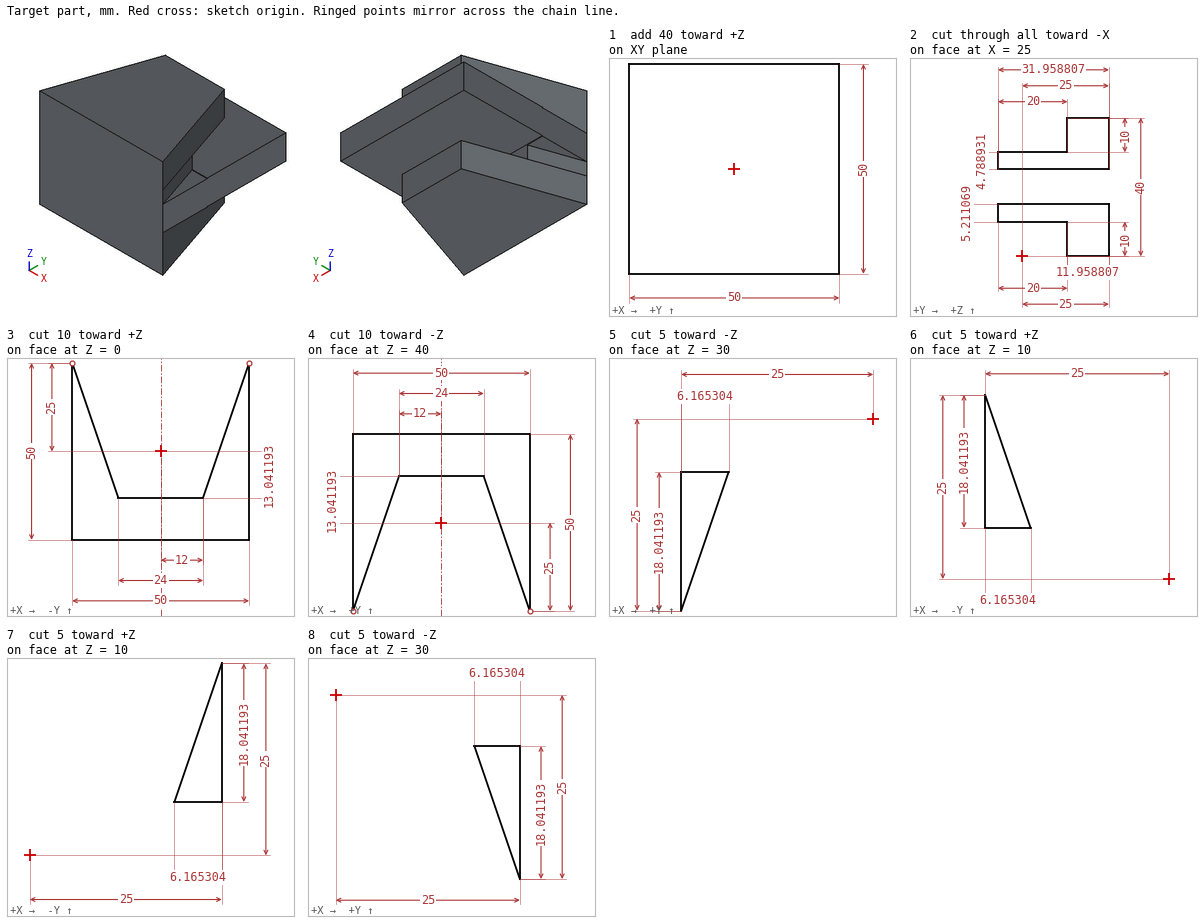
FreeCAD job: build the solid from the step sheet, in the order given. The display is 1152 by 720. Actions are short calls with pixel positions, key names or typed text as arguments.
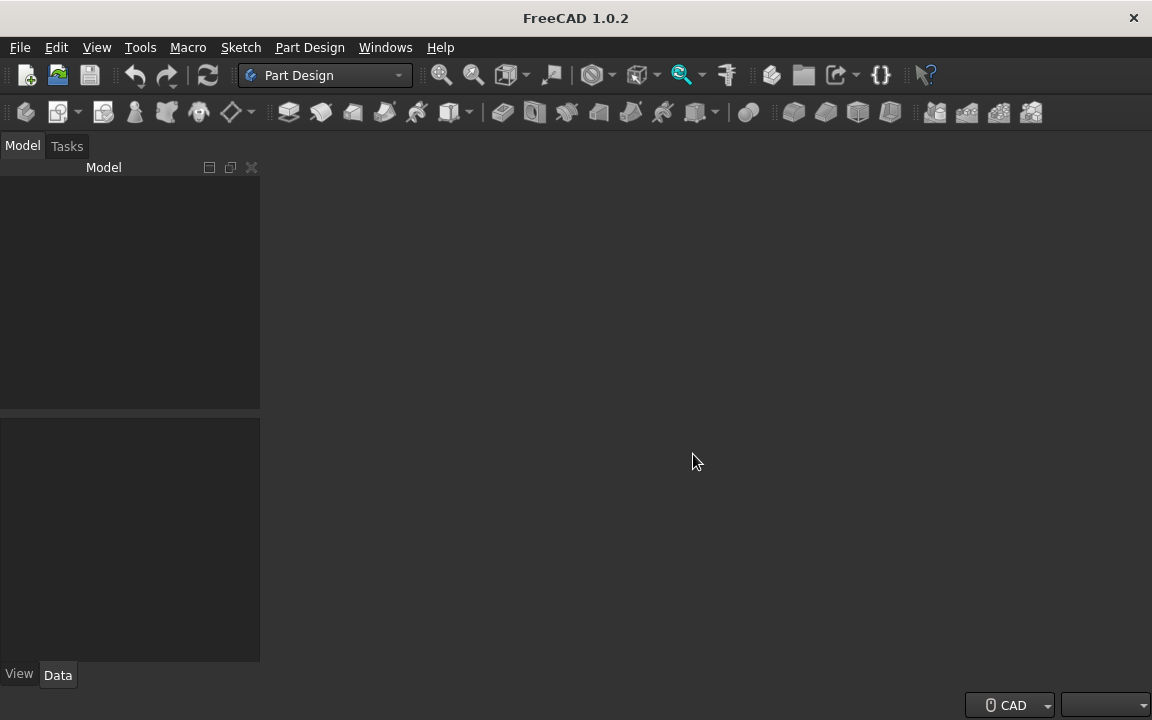
key(ctrl+n)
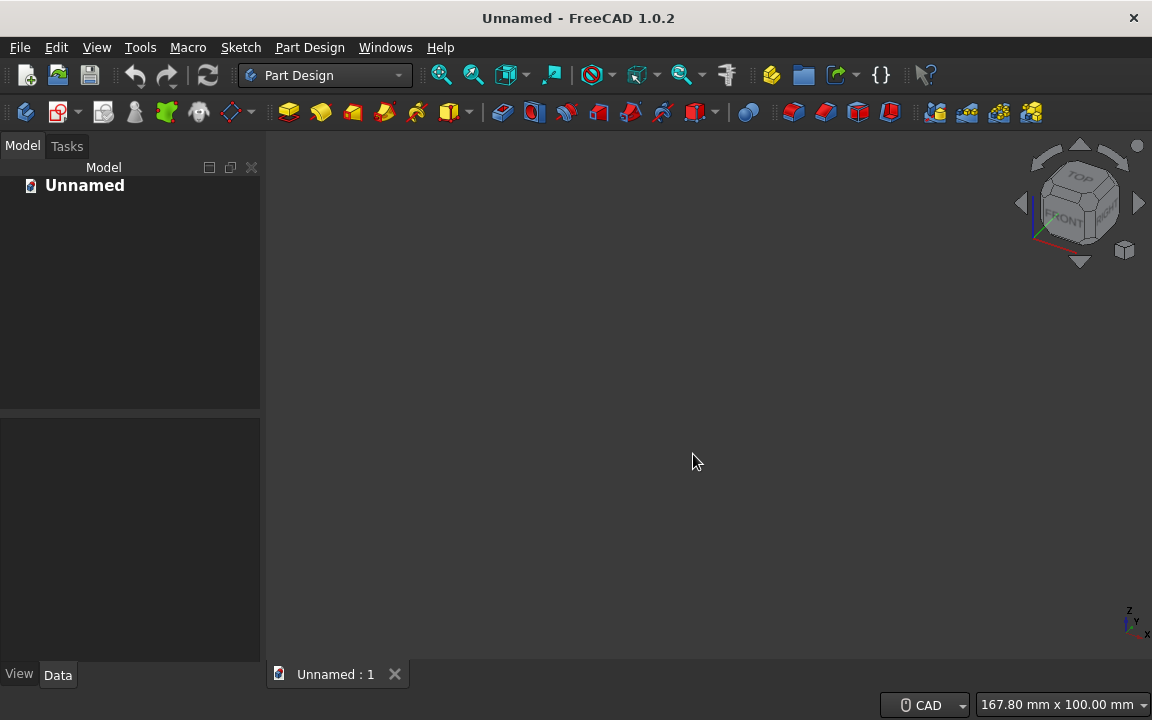
click(58, 112)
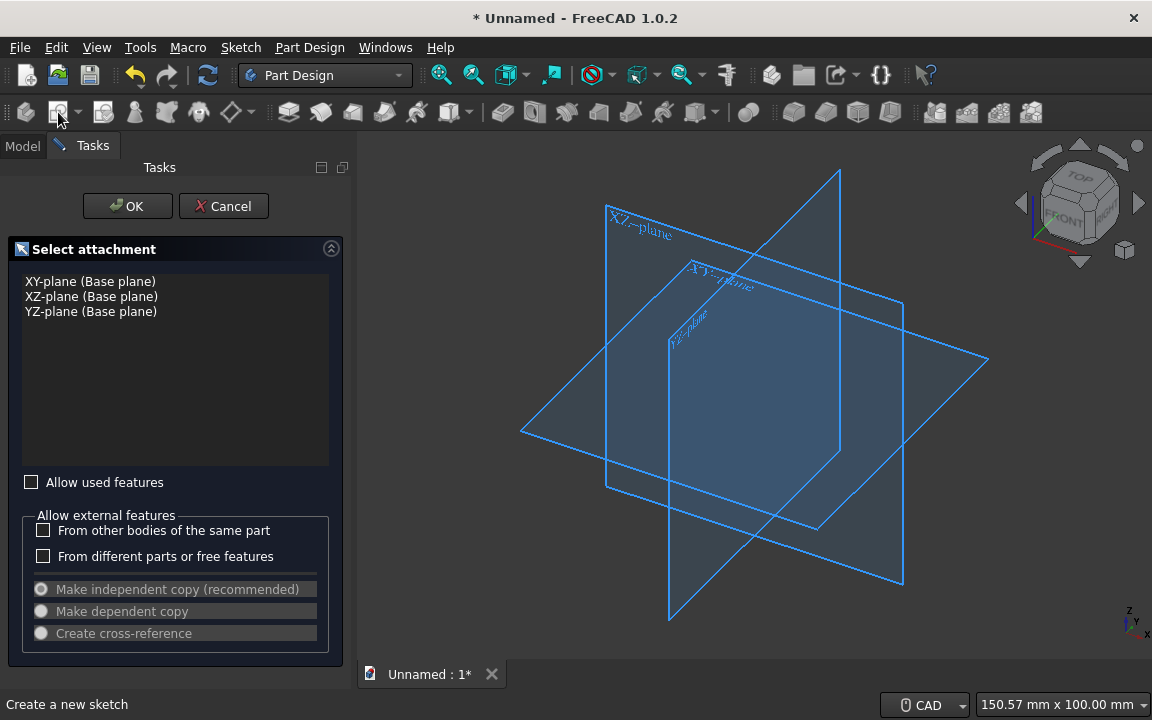
click(82, 282)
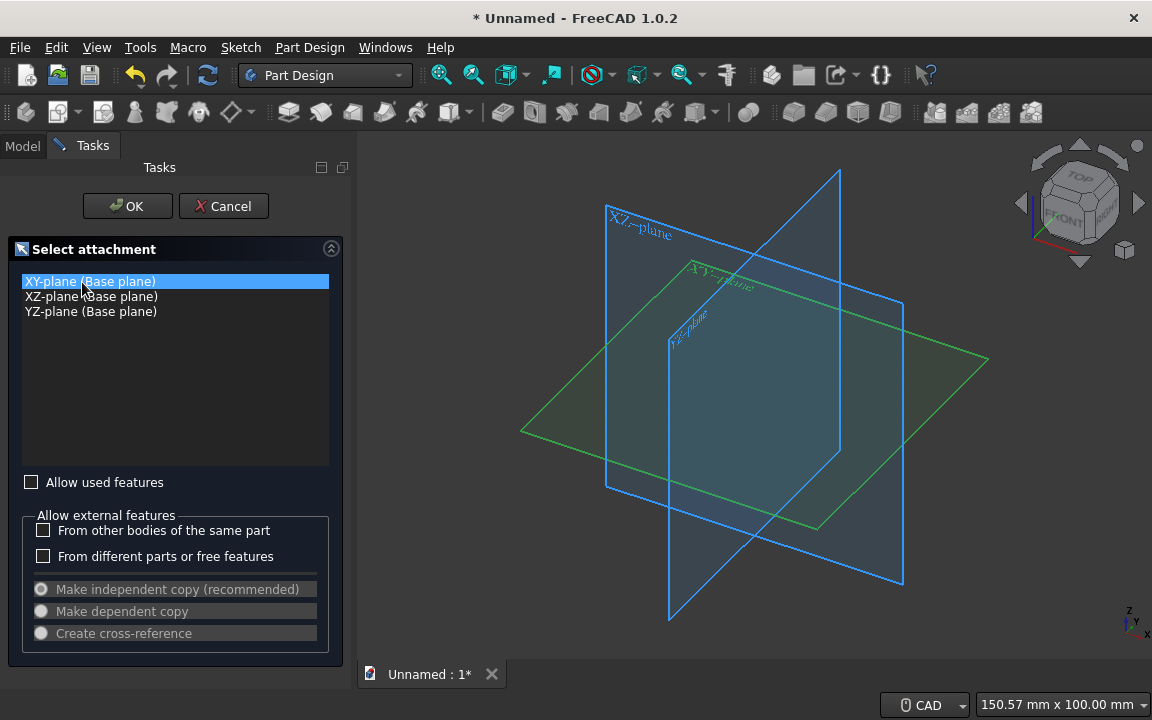
click(128, 206)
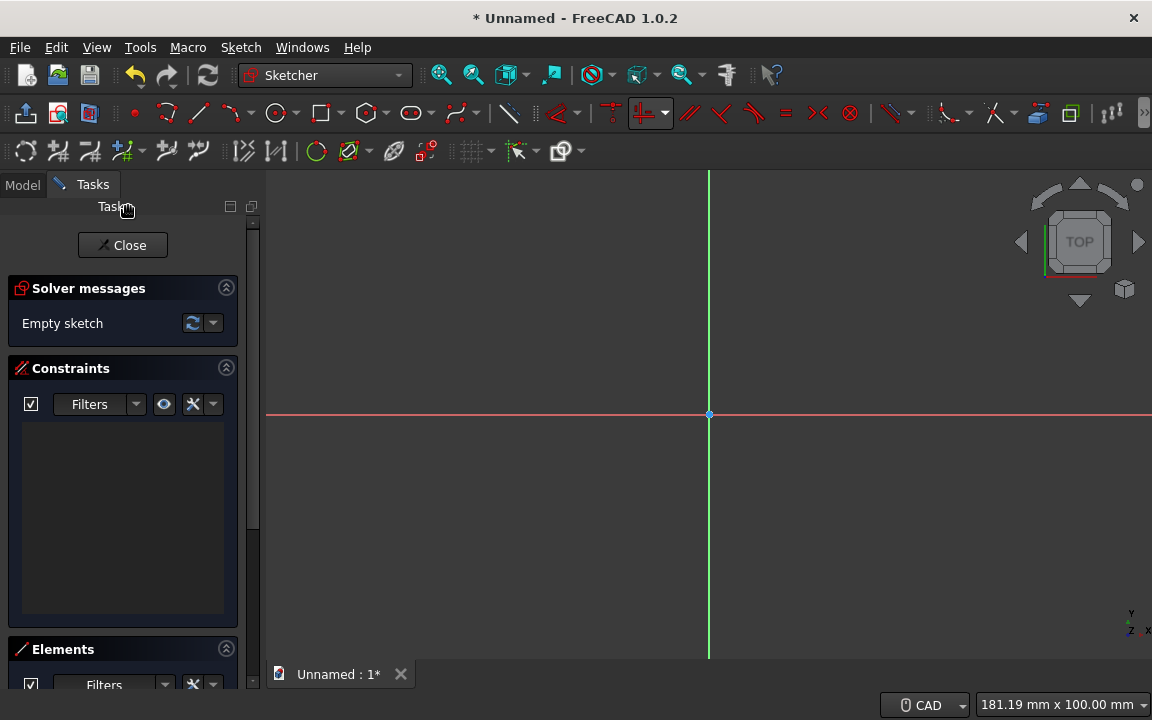
key(g)
key(v)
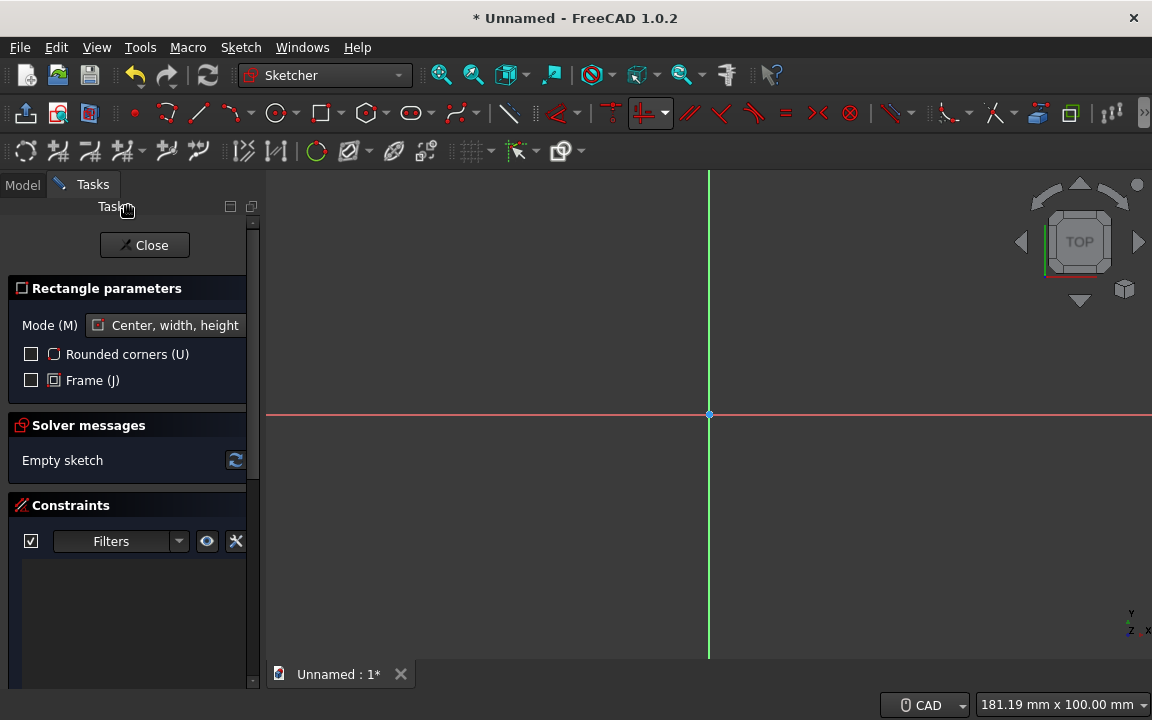
click(709, 414)
click(831, 292)
key(Escape)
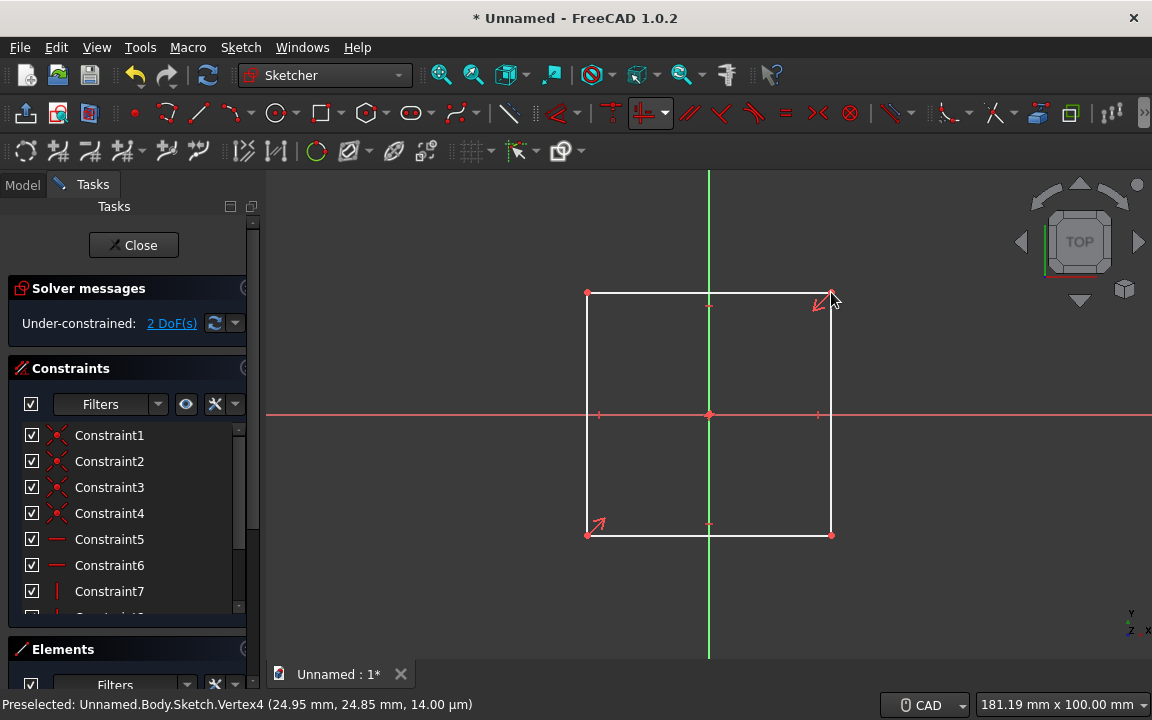
click(660, 536)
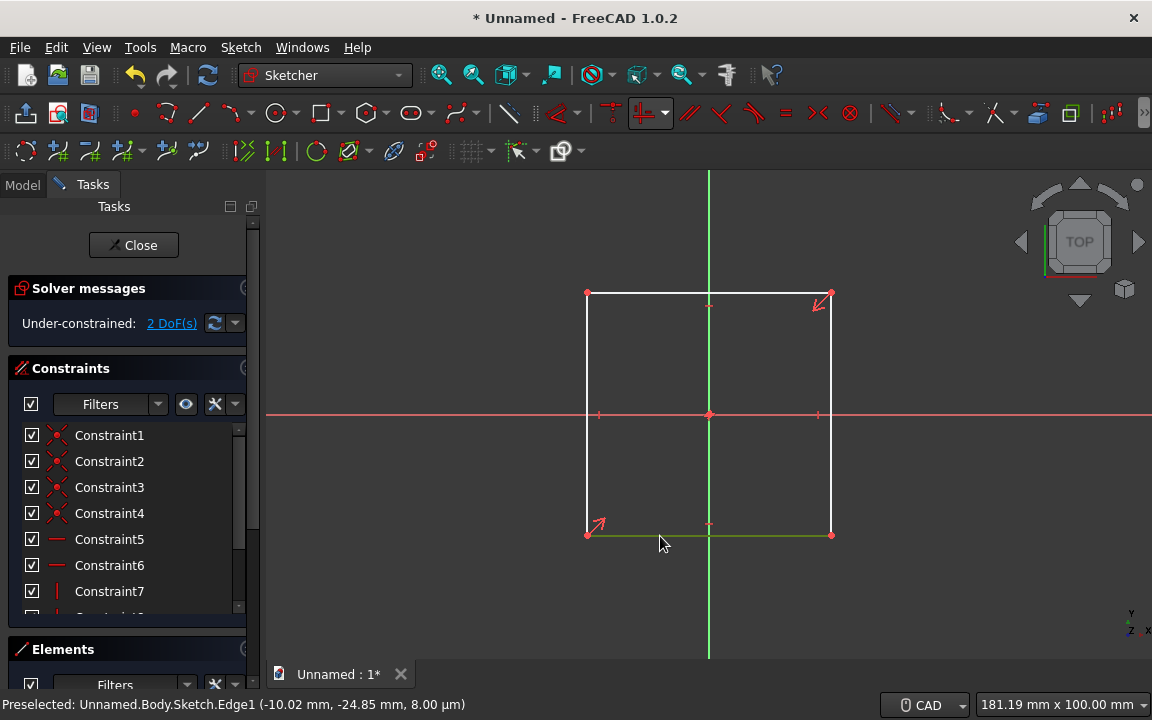
key(l)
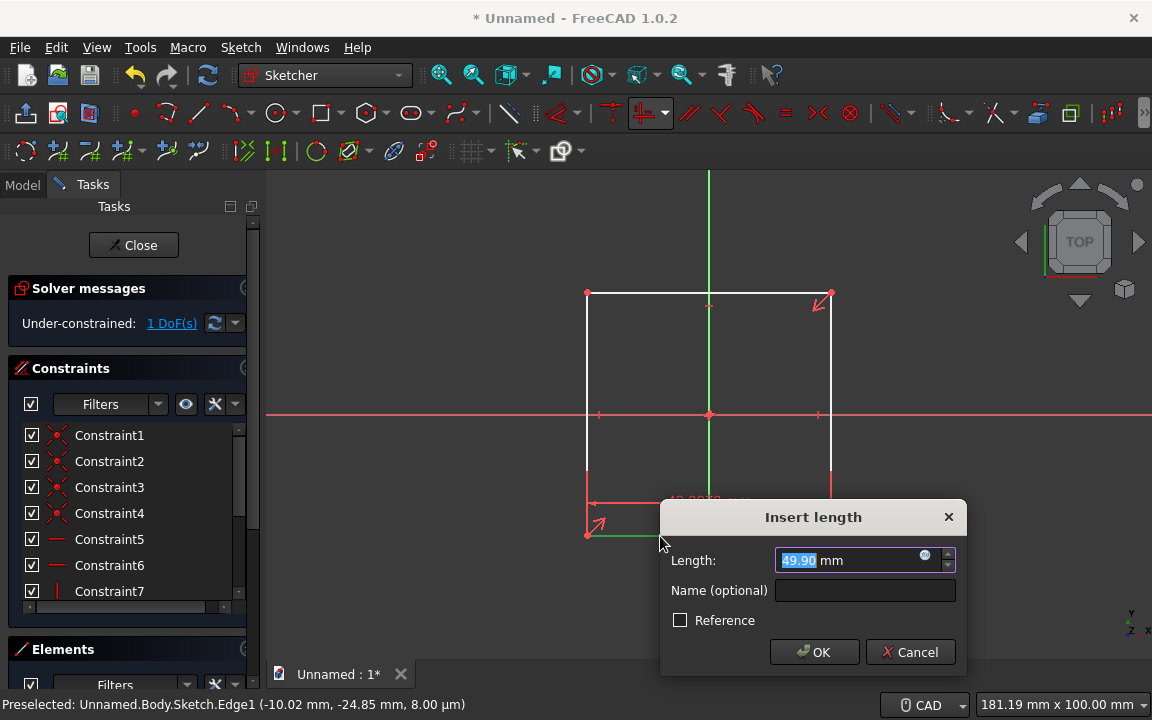
text(50)
key(Return)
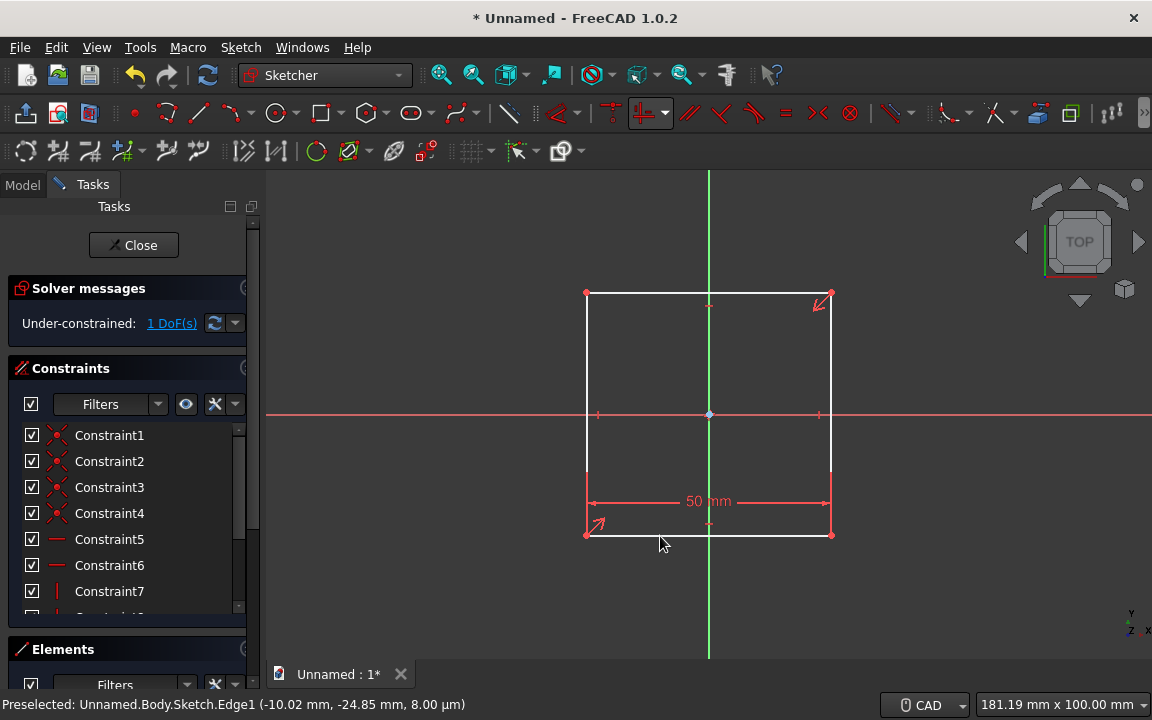
click(831, 463)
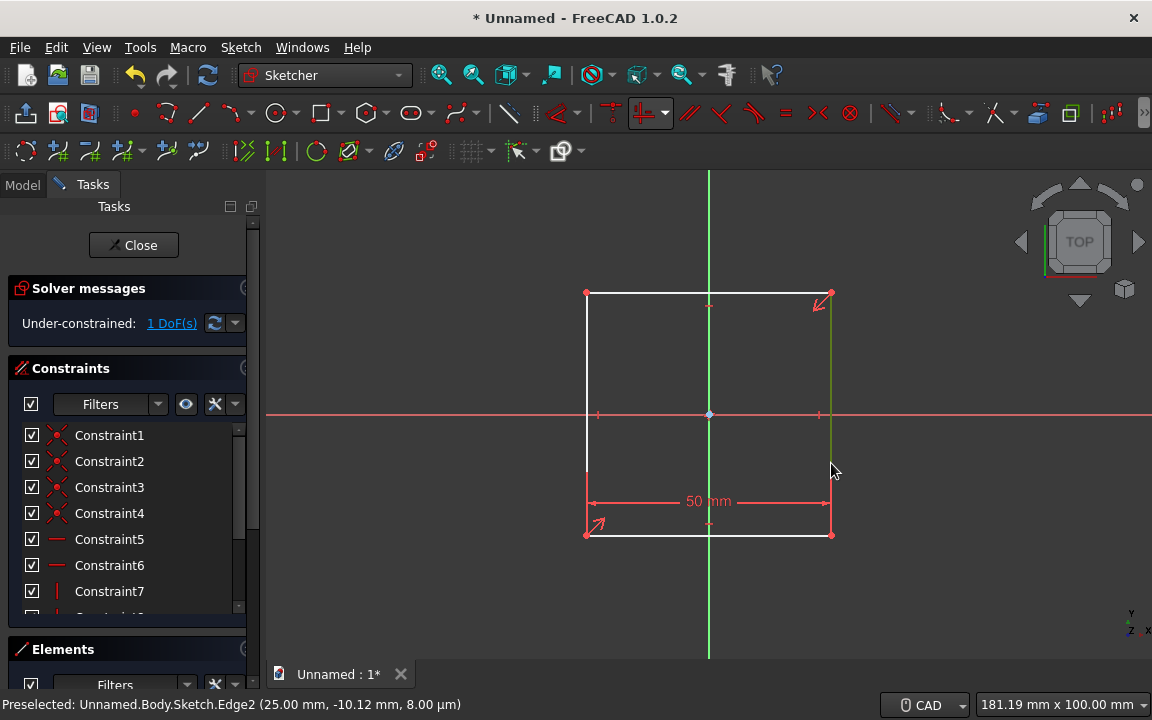
key(i)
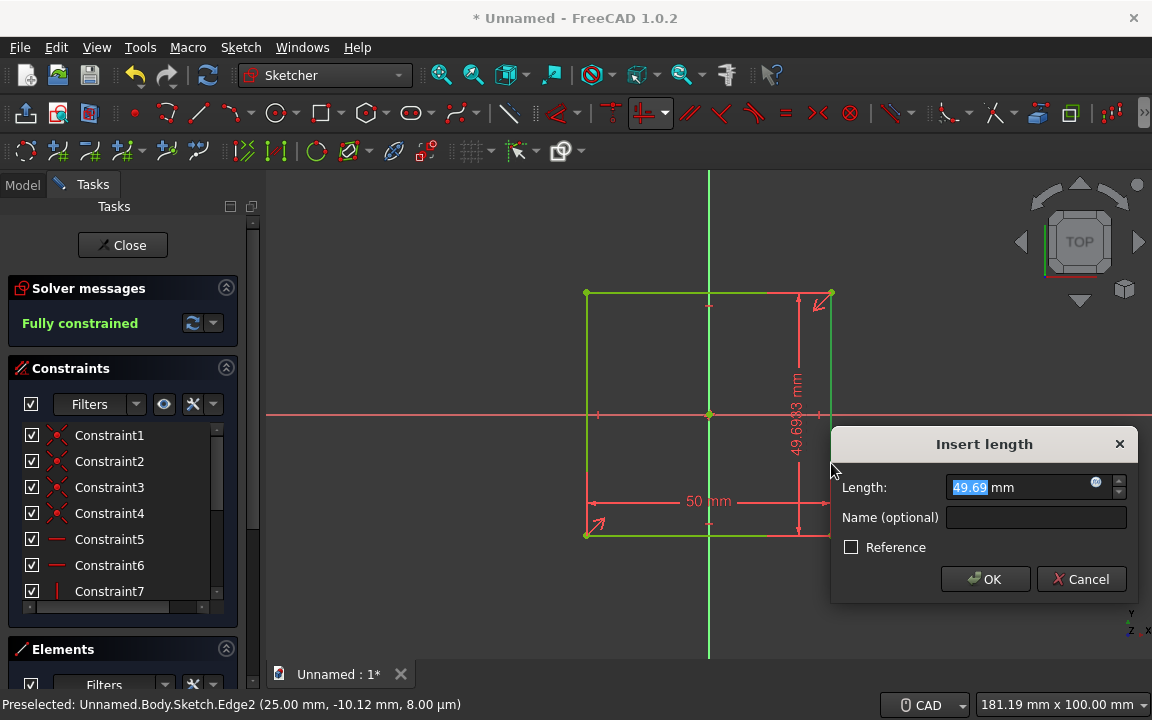
text(50)
key(Return)